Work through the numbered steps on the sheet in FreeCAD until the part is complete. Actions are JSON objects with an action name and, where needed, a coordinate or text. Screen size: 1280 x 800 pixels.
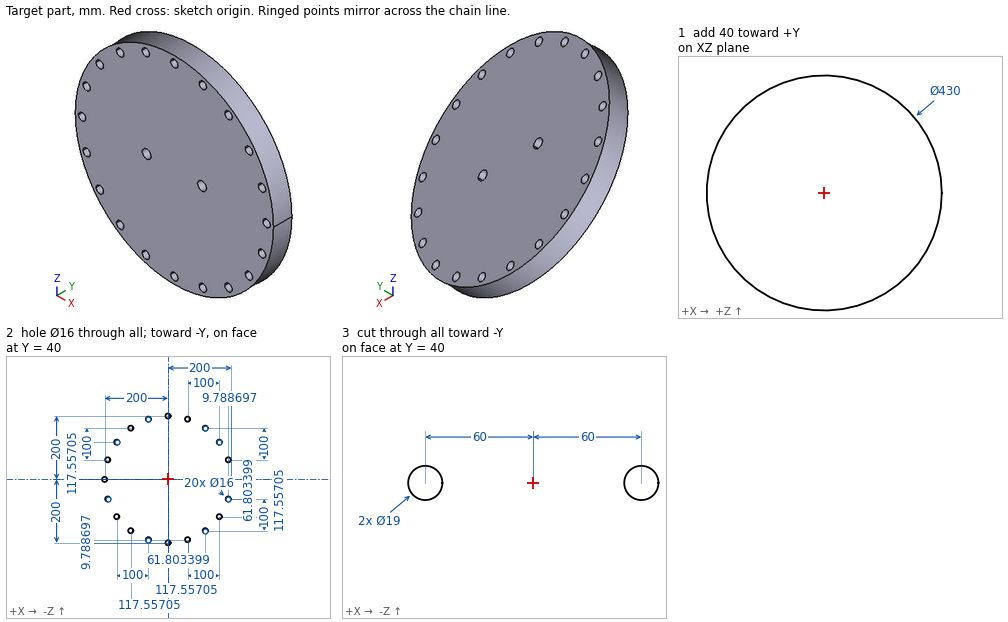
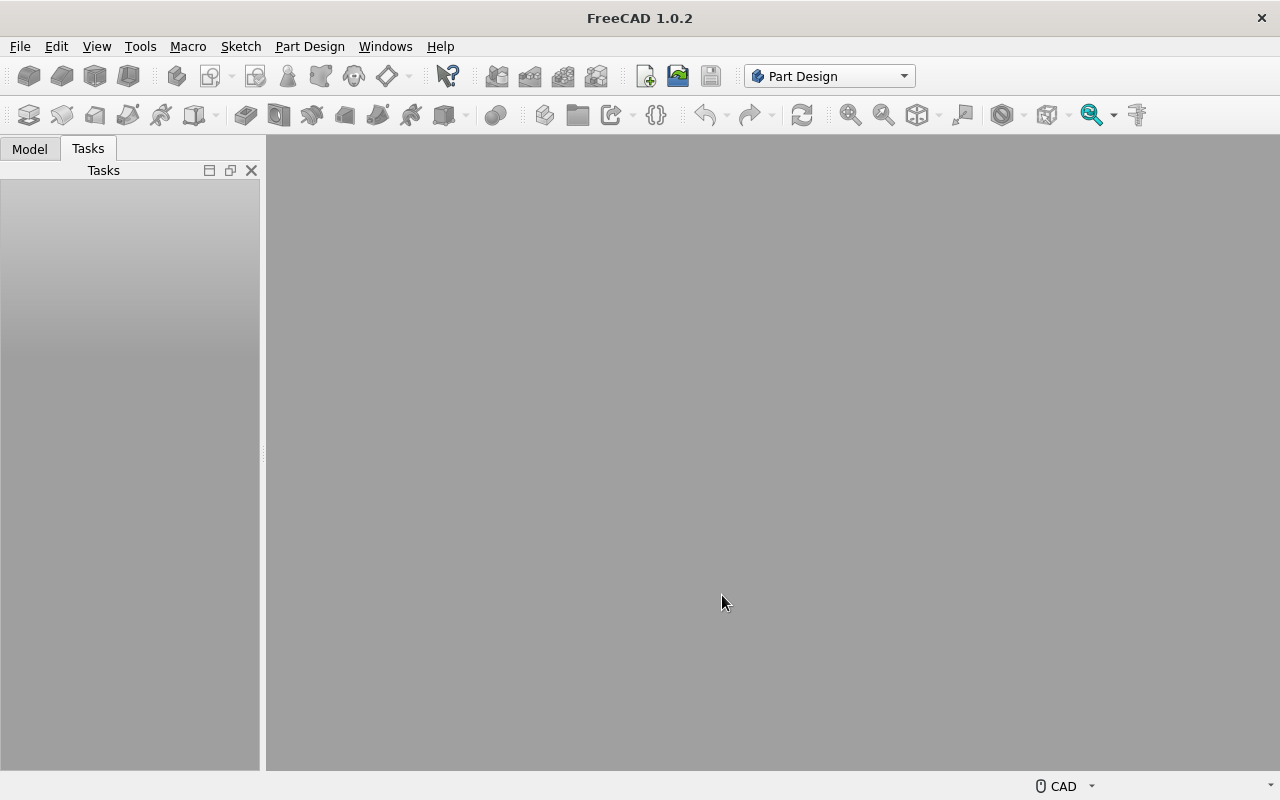
{"action": "key", "text": "ctrl+n"}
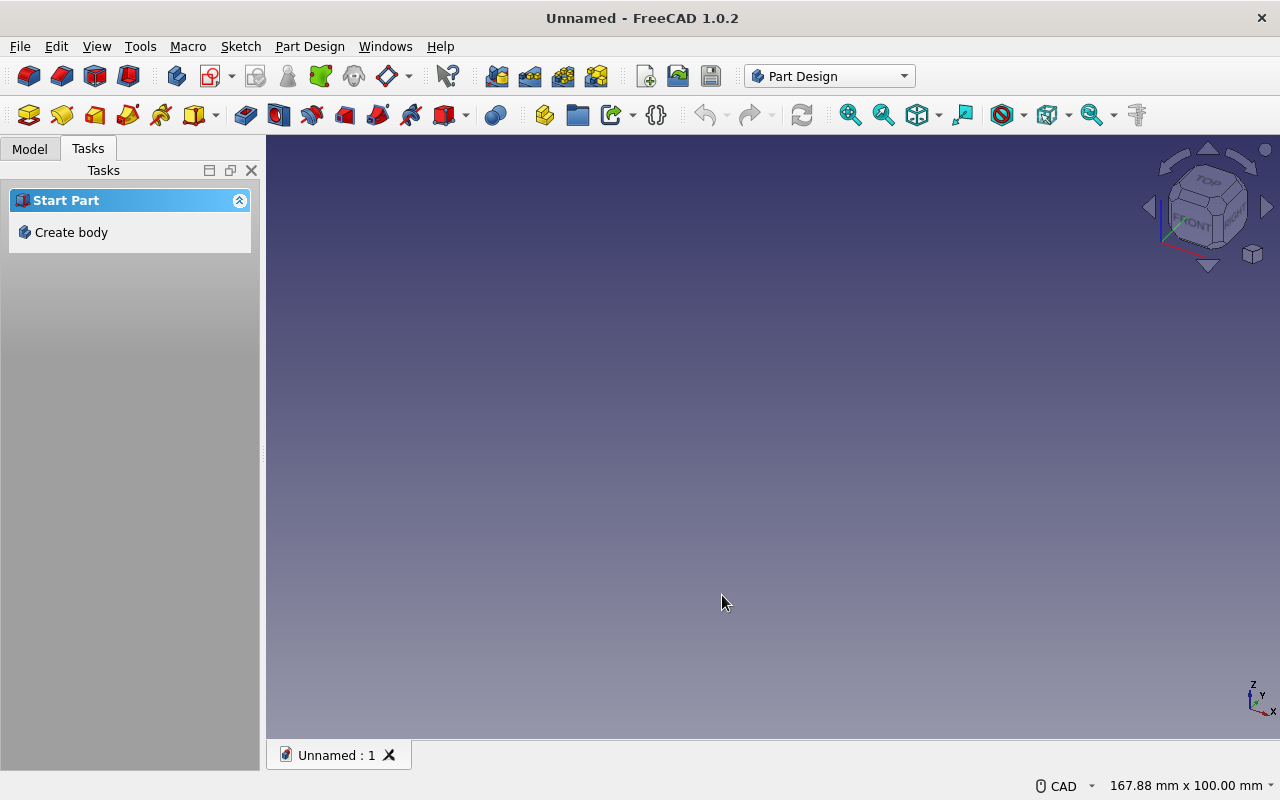
{"action": "left_click", "coordinate": [210, 76]}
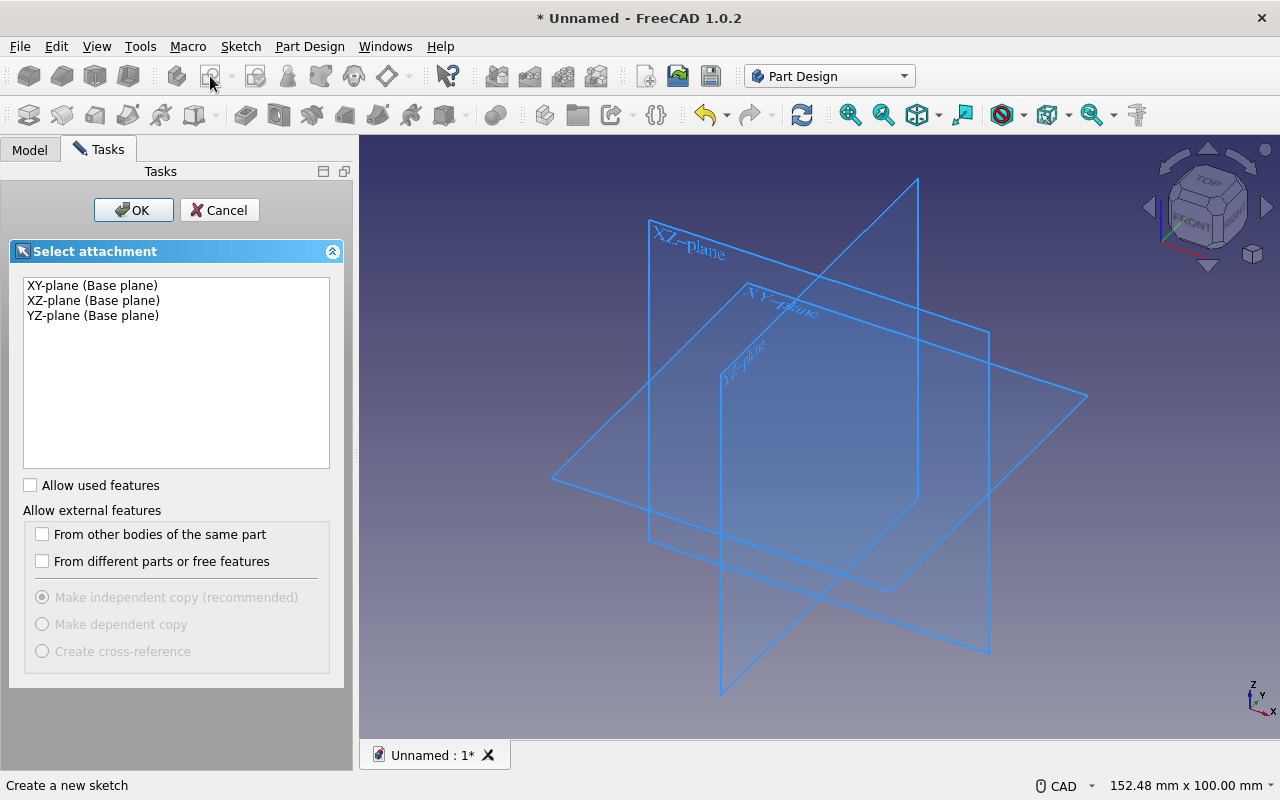
{"action": "left_click", "coordinate": [84, 300]}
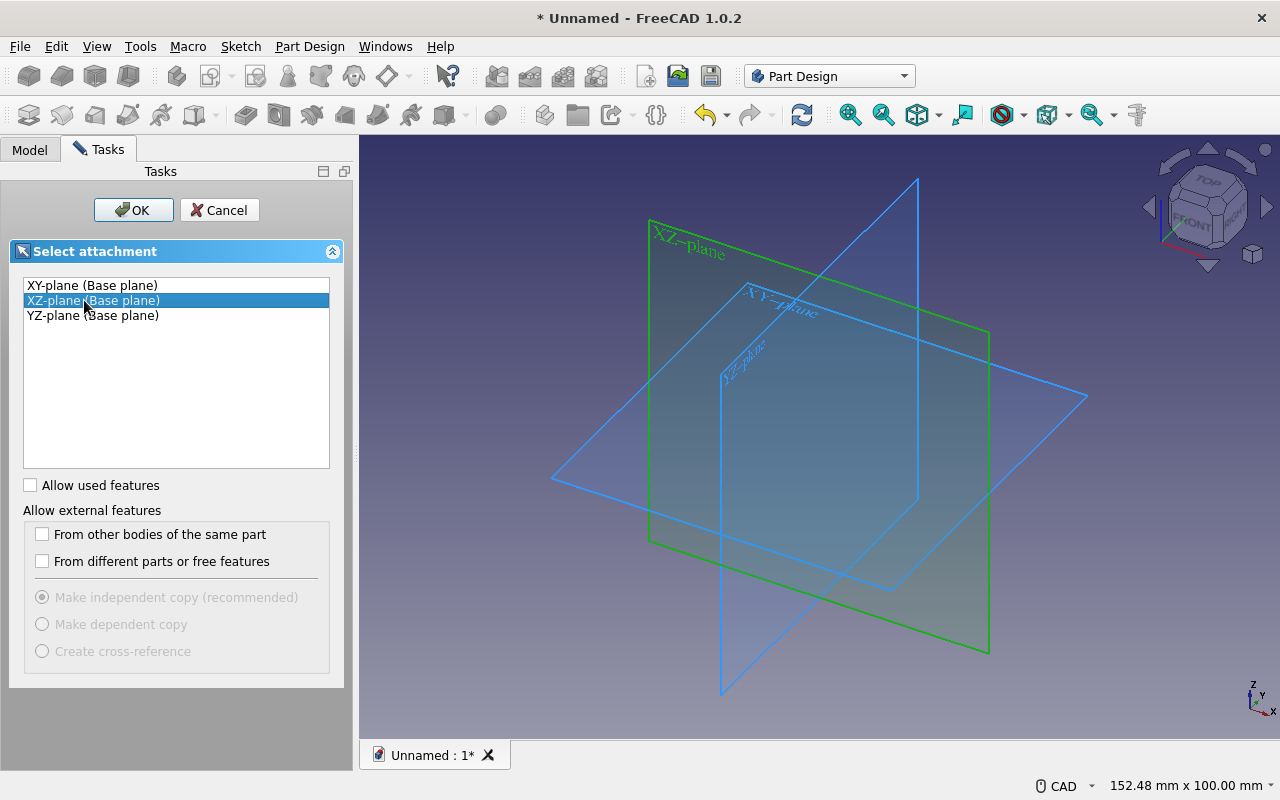
{"action": "left_click", "coordinate": [134, 210]}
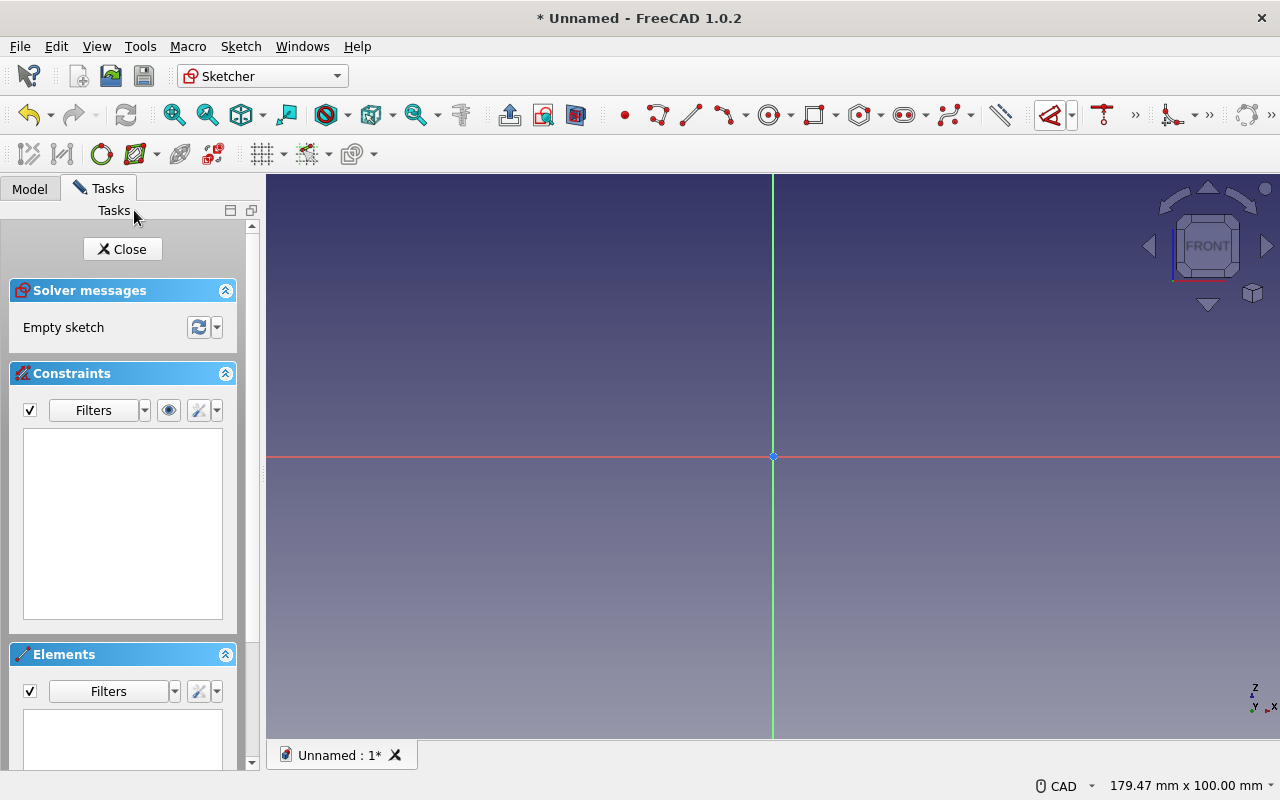
{"action": "scroll", "coordinate": [694, 457], "scroll_direction": "down", "scroll_amount": 10}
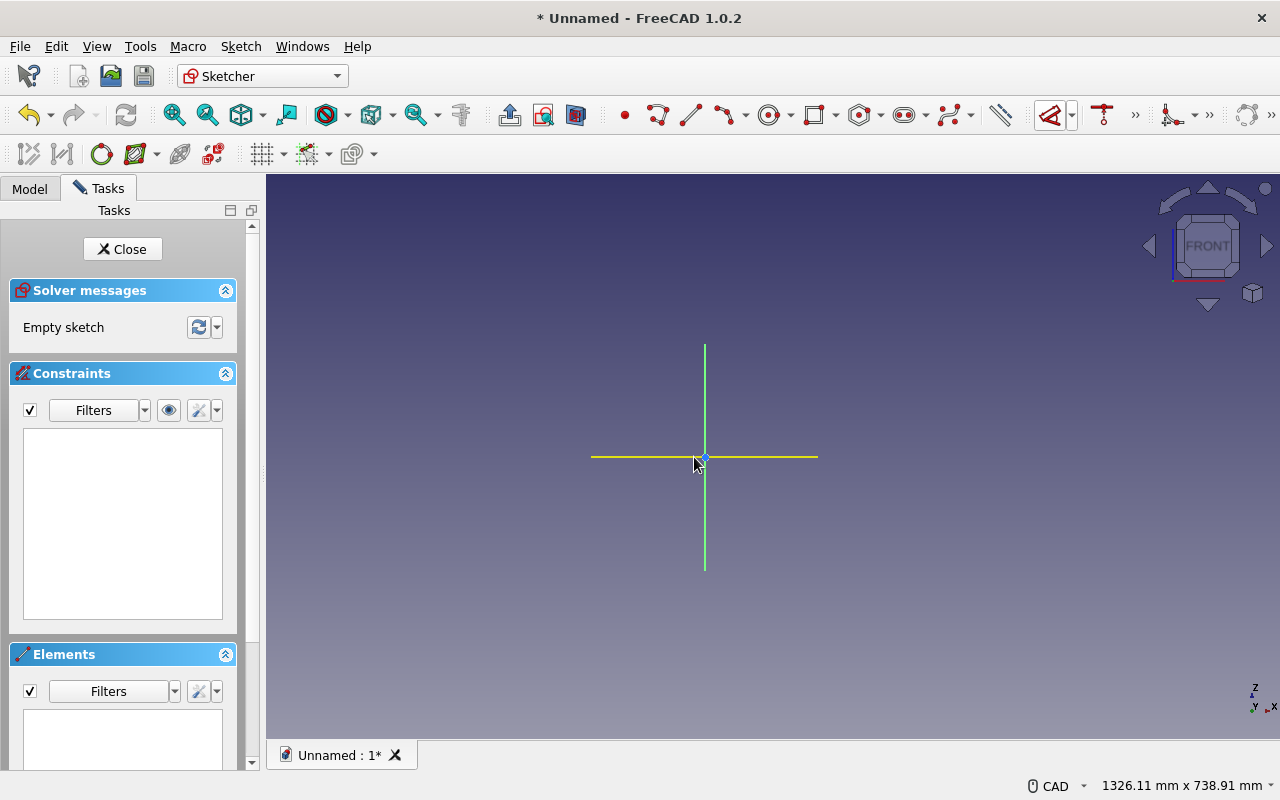
{"action": "key", "text": "g c"}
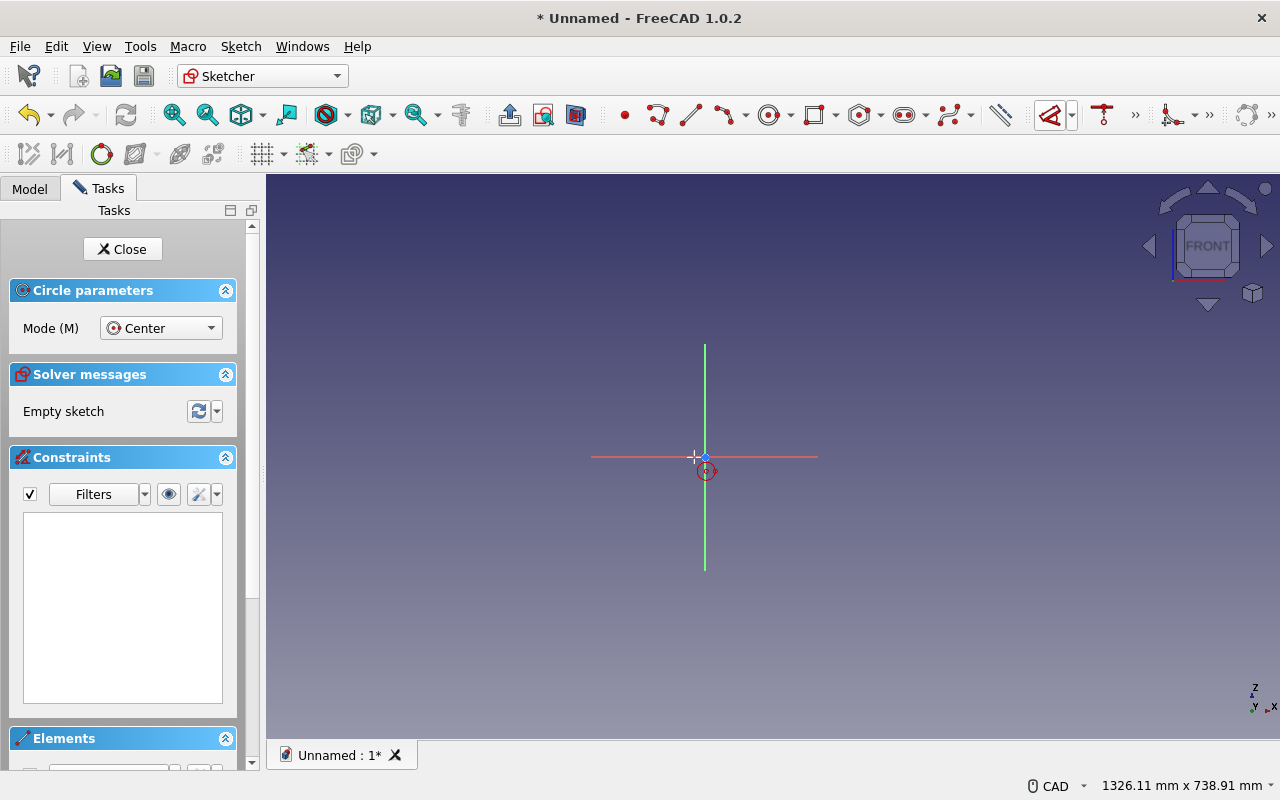
{"action": "left_click", "coordinate": [705, 457]}
{"action": "left_click", "coordinate": [821, 341]}
{"action": "key", "text": "Escape"}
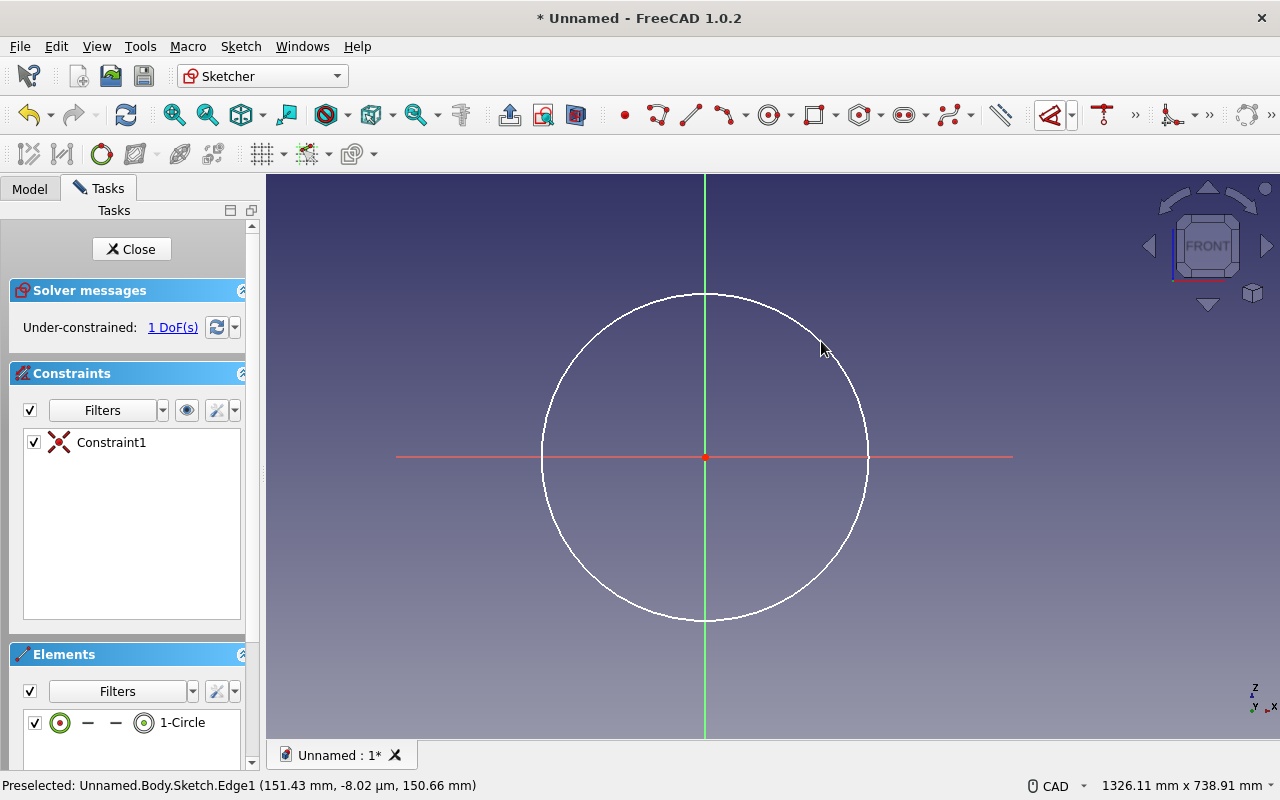
{"action": "key", "text": "d"}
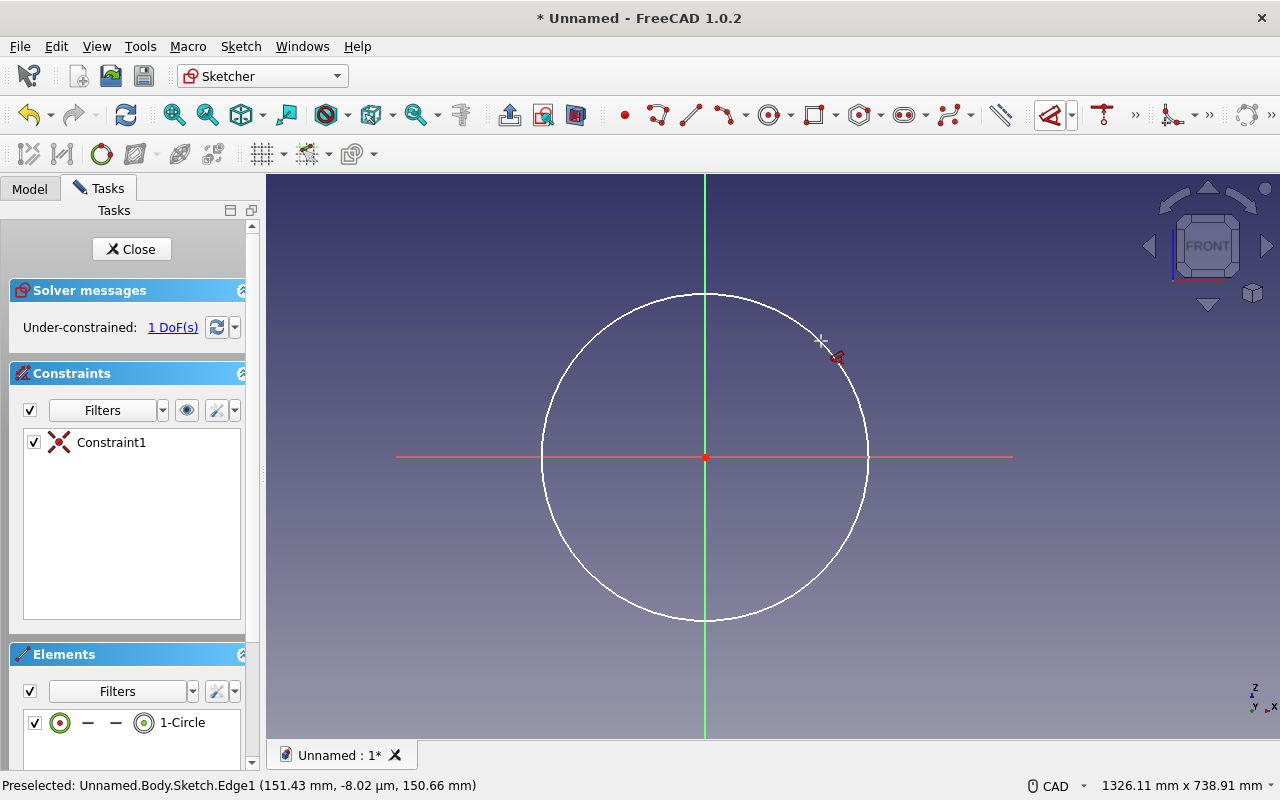
{"action": "left_click", "coordinate": [820, 341]}
{"action": "left_click", "coordinate": [842, 318]}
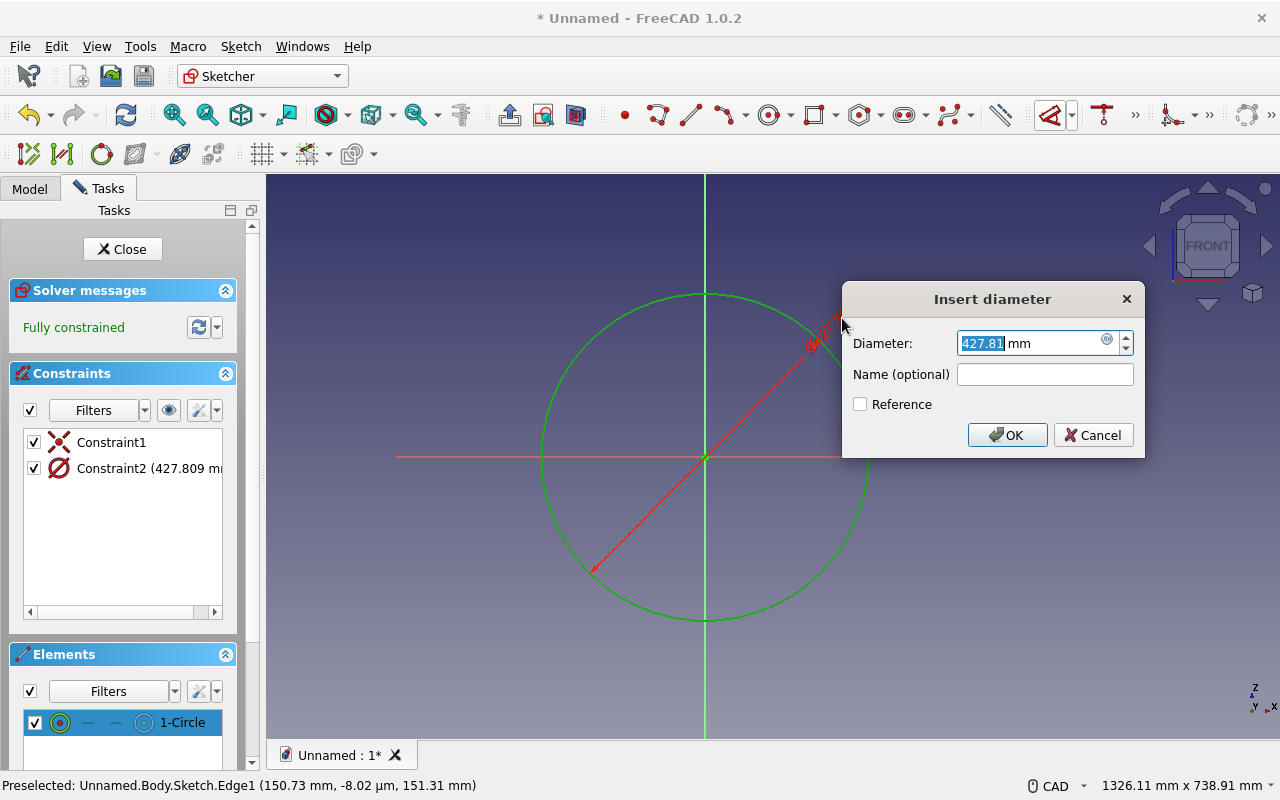
{"action": "type", "text": "430"}
{"action": "key", "text": "Return"}
{"action": "key", "text": "Escape"}